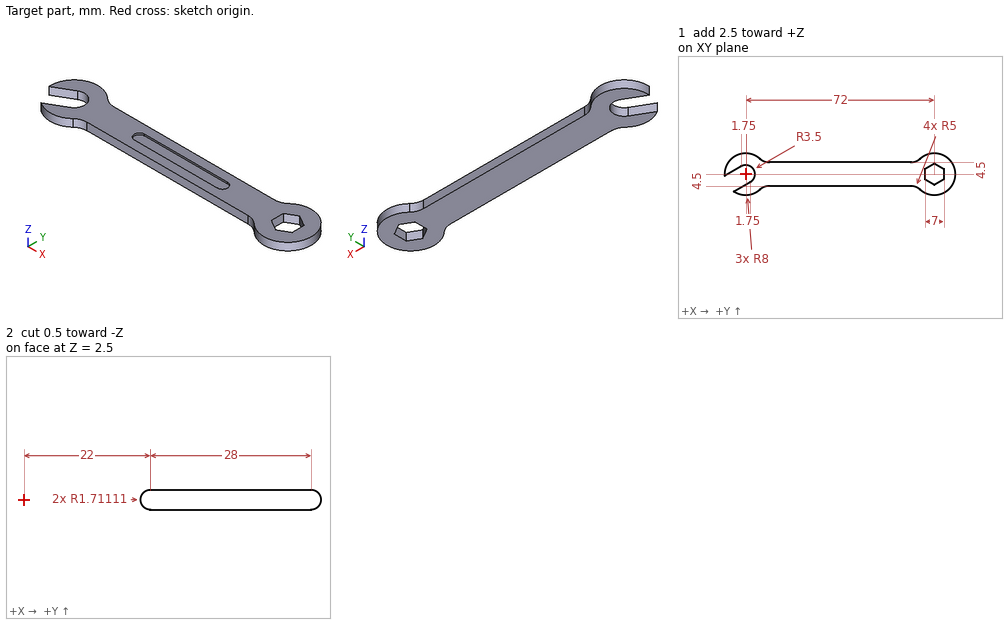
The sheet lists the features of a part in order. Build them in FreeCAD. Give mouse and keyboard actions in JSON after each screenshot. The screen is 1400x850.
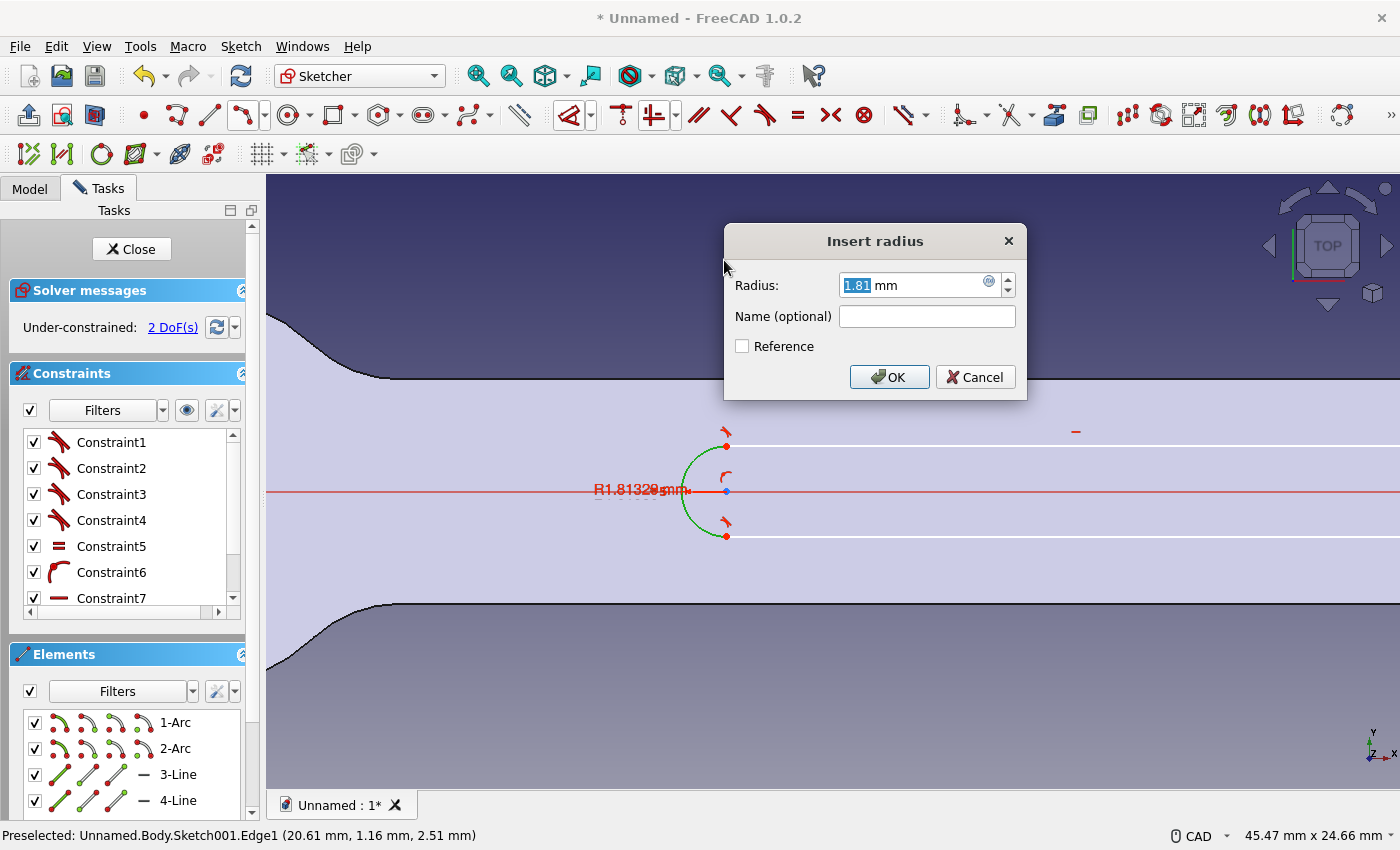
{"action": "type", "text": "1.71111"}
{"action": "key", "text": "Return"}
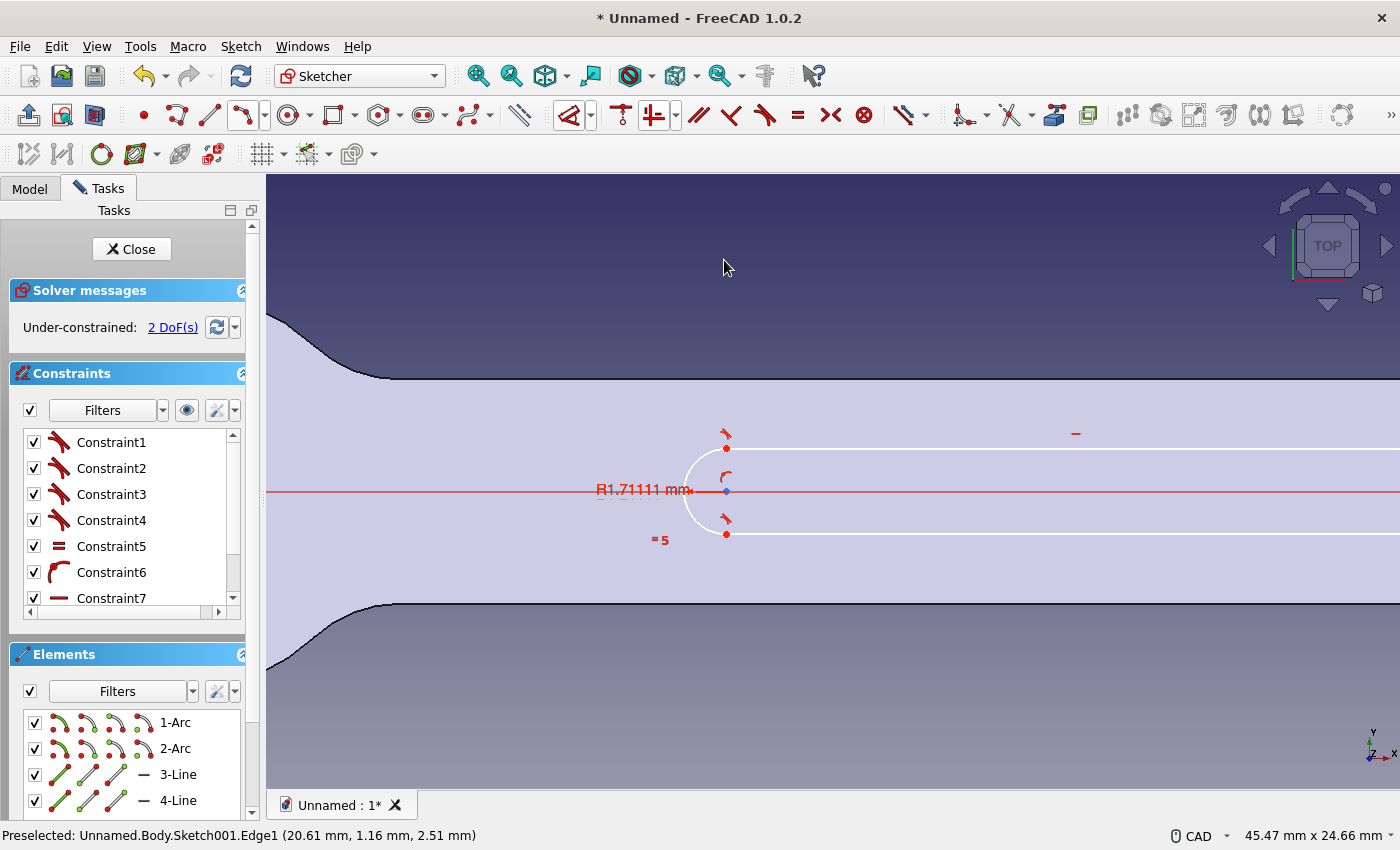
{"action": "left_click", "coordinate": [936, 449]}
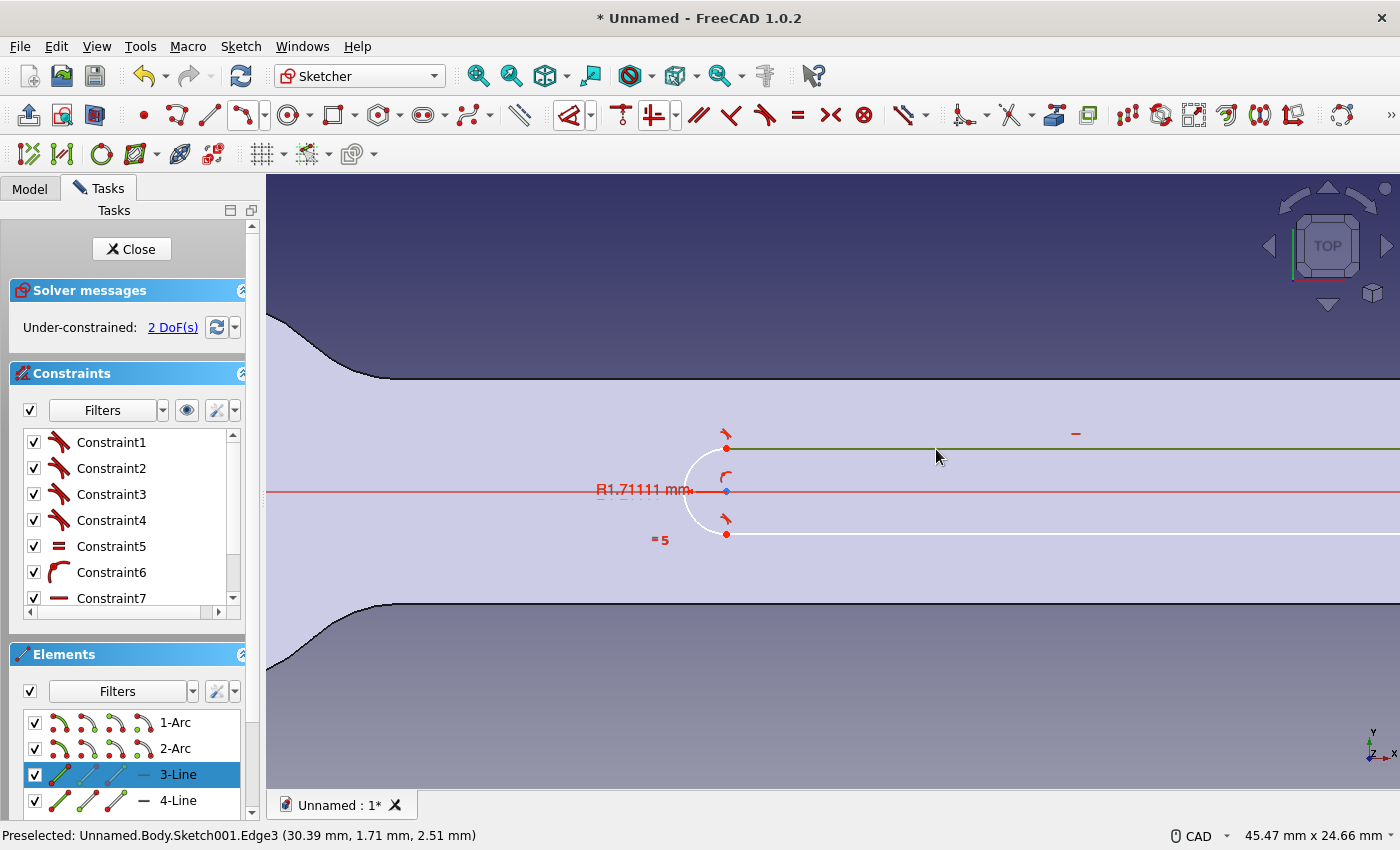
{"action": "left_click", "coordinate": [590, 116]}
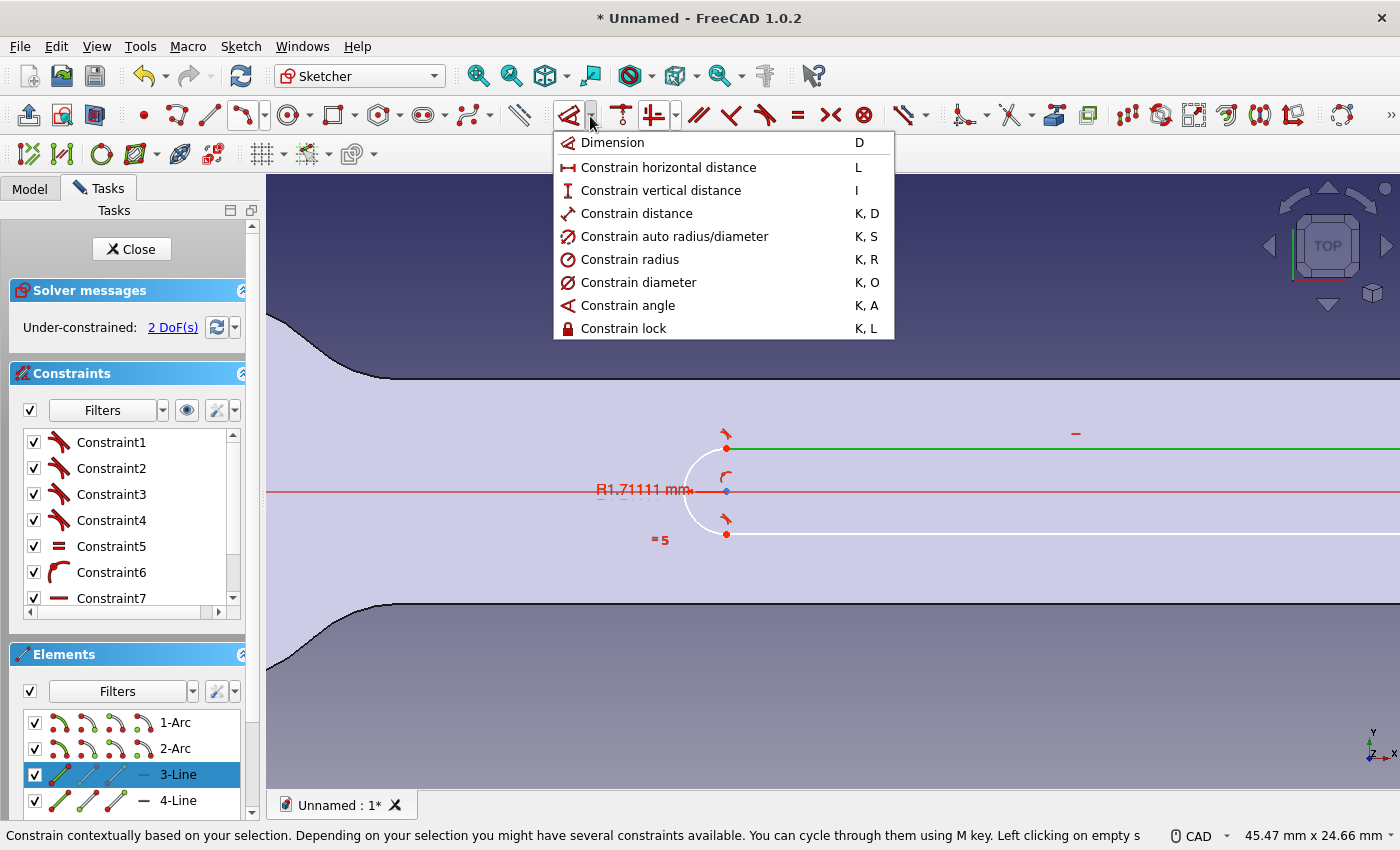
{"action": "left_click", "coordinate": [724, 168]}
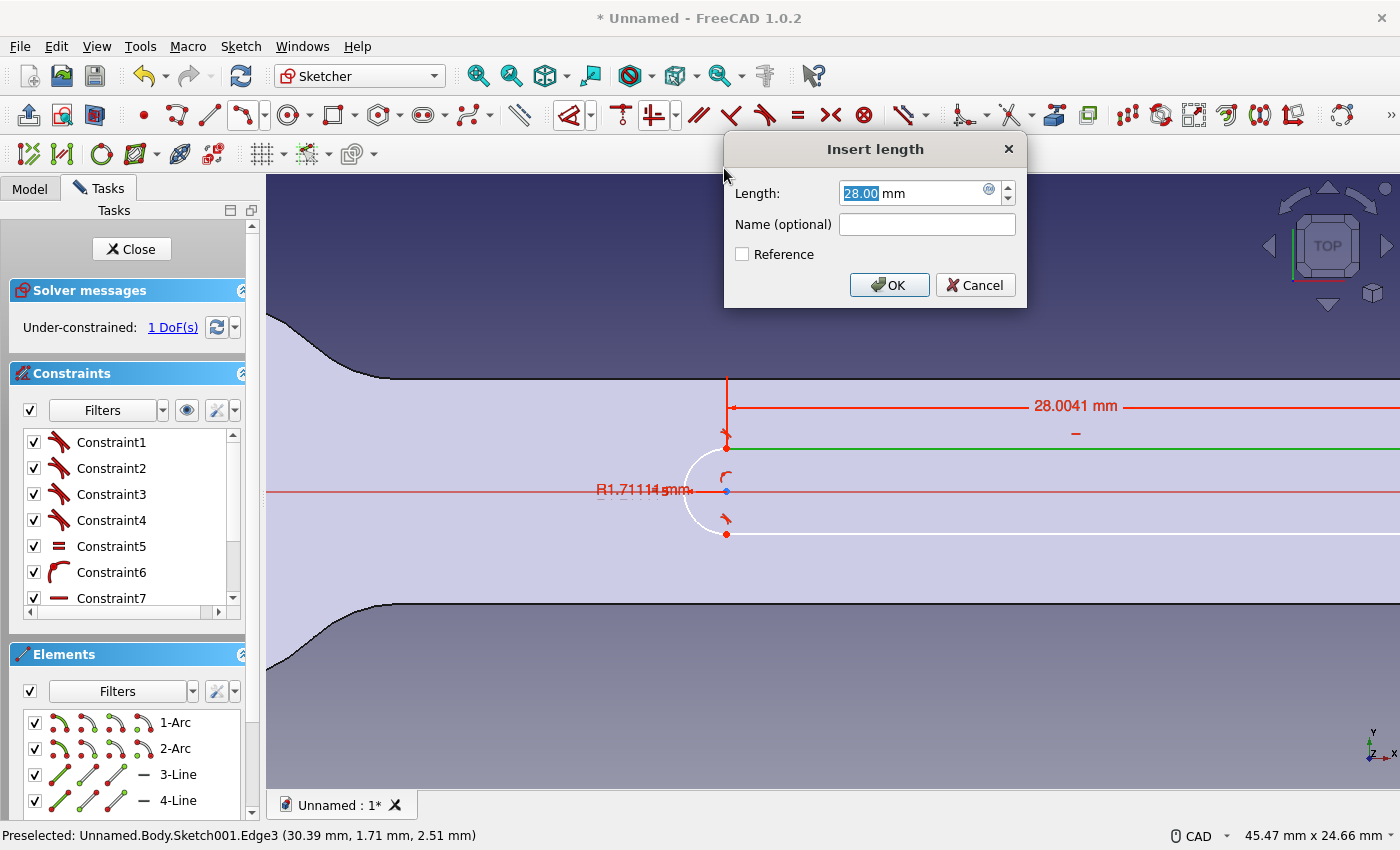
{"action": "type", "text": "28"}
{"action": "key", "text": "Return"}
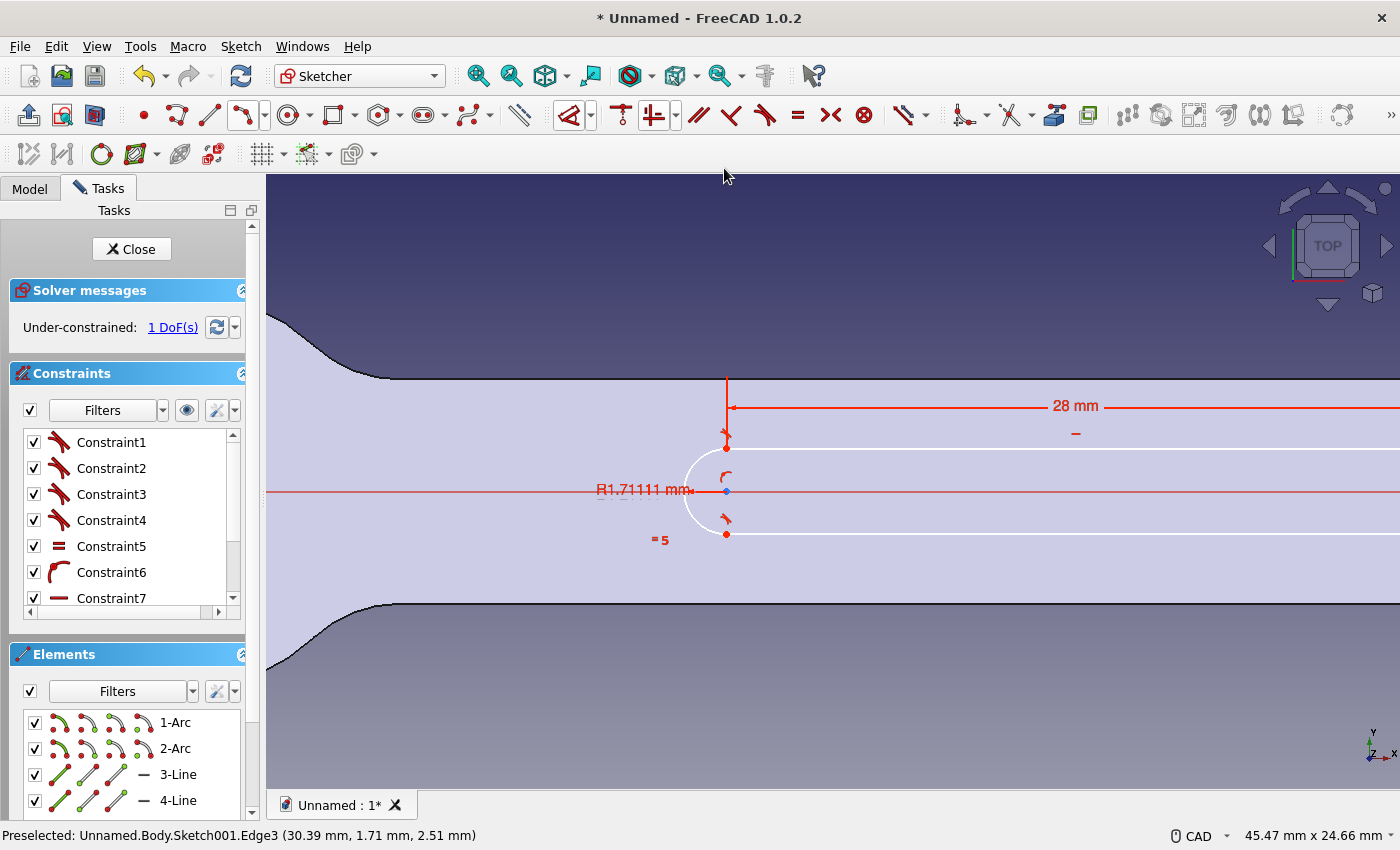
{"action": "left_click", "coordinate": [727, 449]}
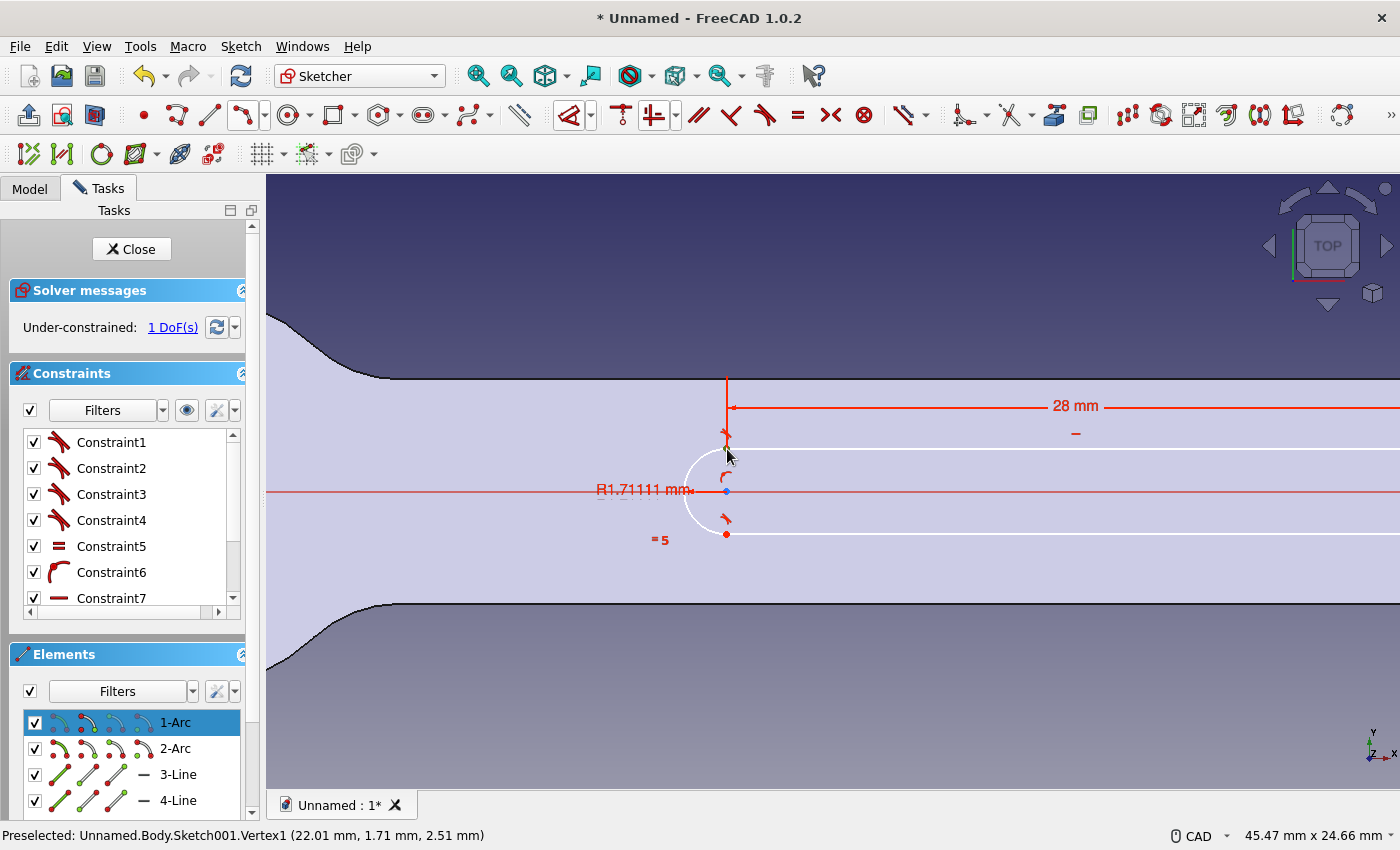
{"action": "left_click", "coordinate": [590, 116]}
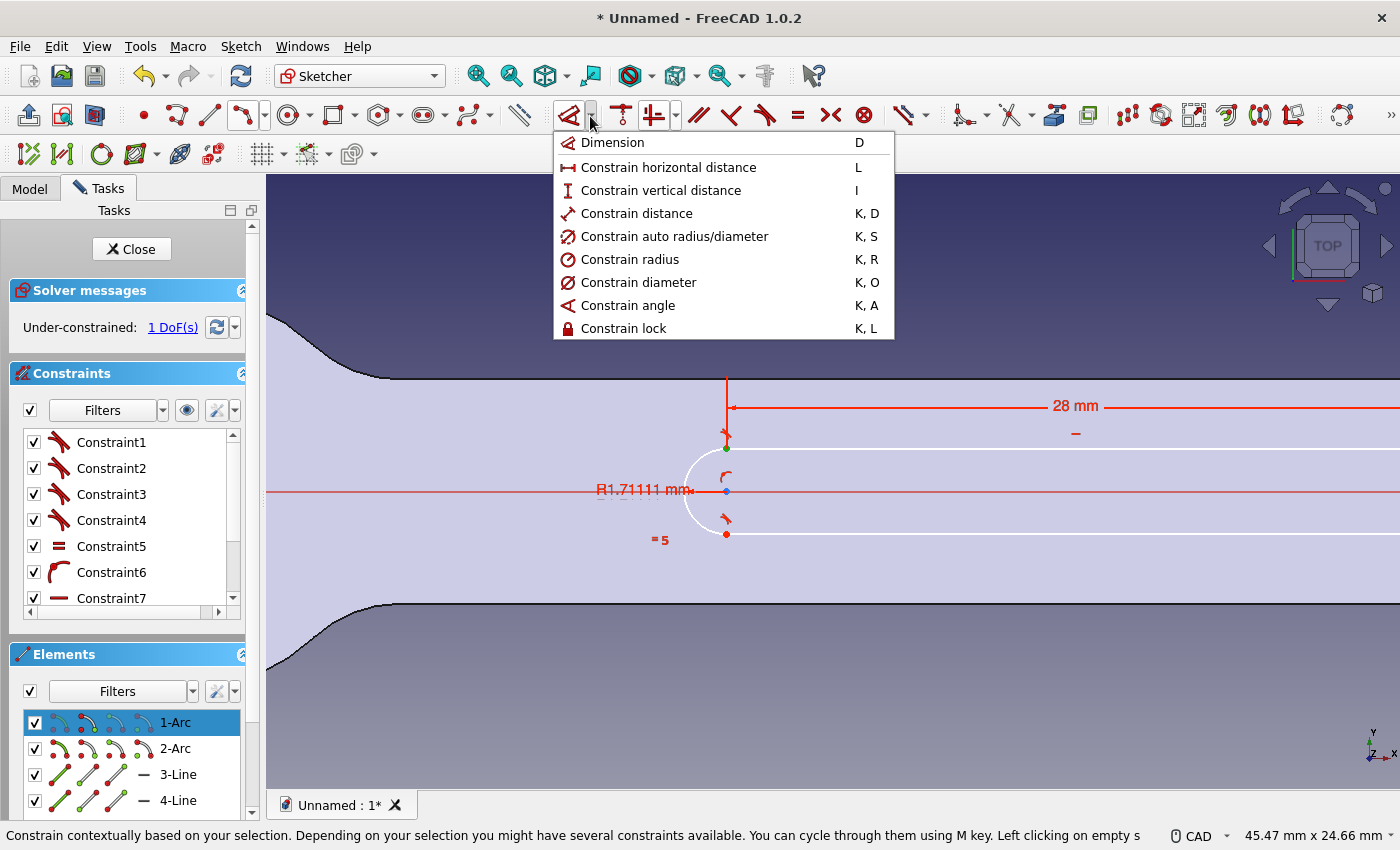
{"action": "left_click", "coordinate": [724, 168]}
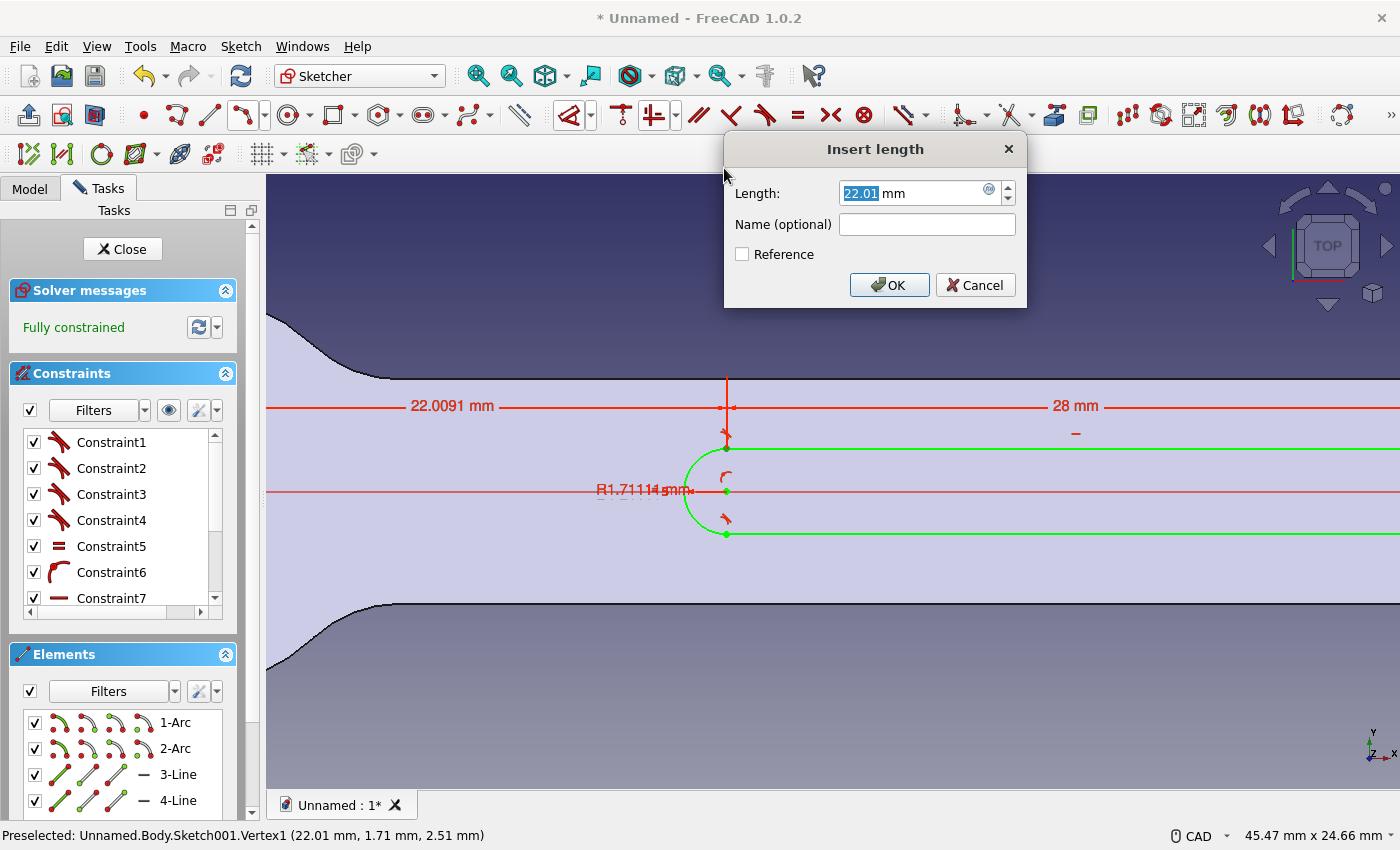
{"action": "type", "text": "22"}
{"action": "key", "text": "Return"}